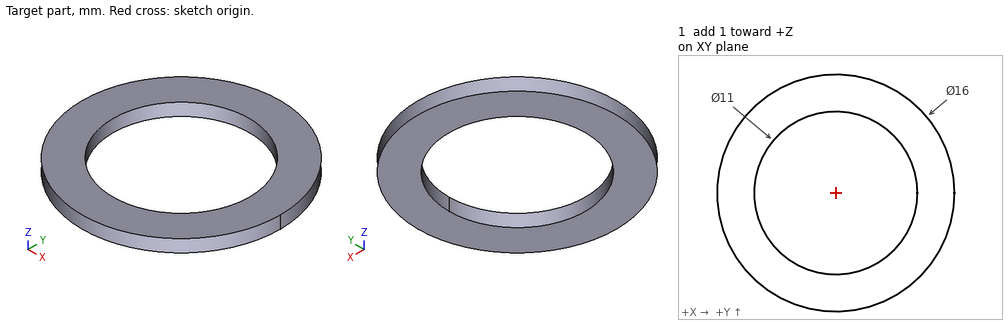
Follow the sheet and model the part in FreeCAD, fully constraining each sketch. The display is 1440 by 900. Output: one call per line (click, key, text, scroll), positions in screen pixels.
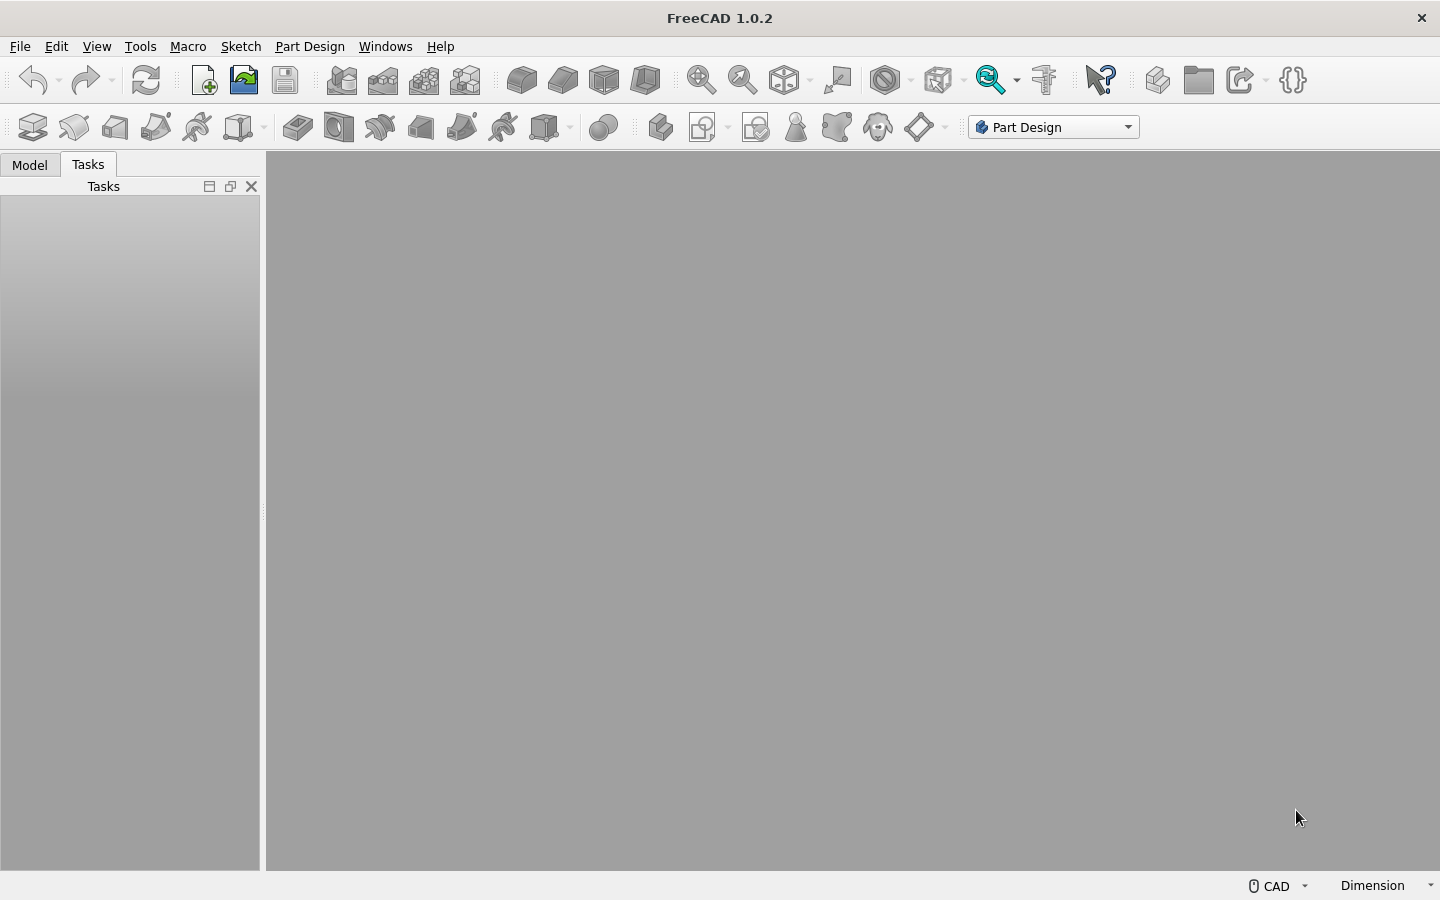
click(203, 80)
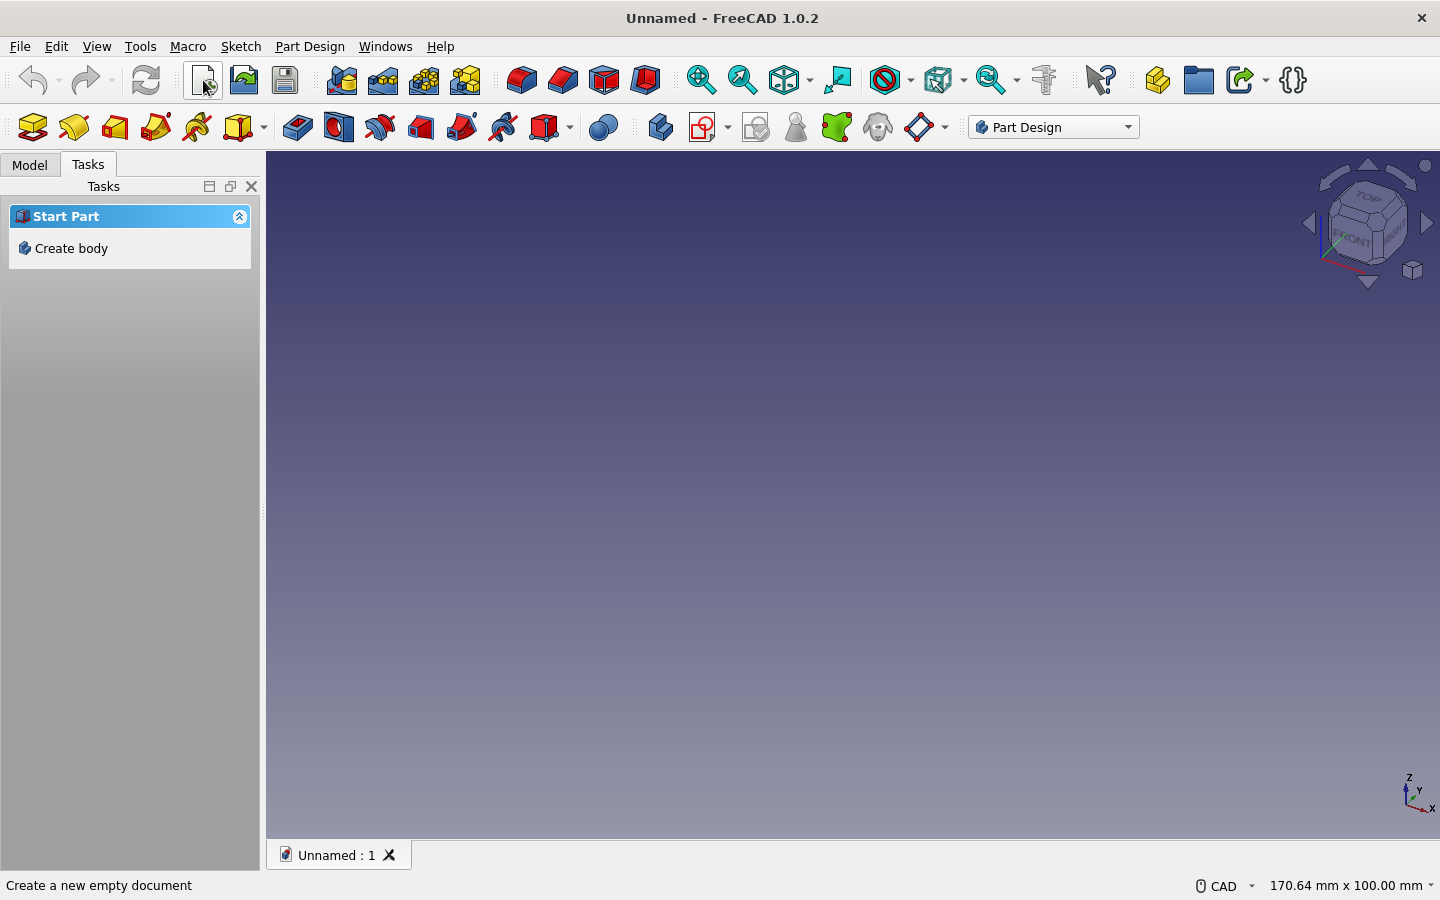
click(702, 128)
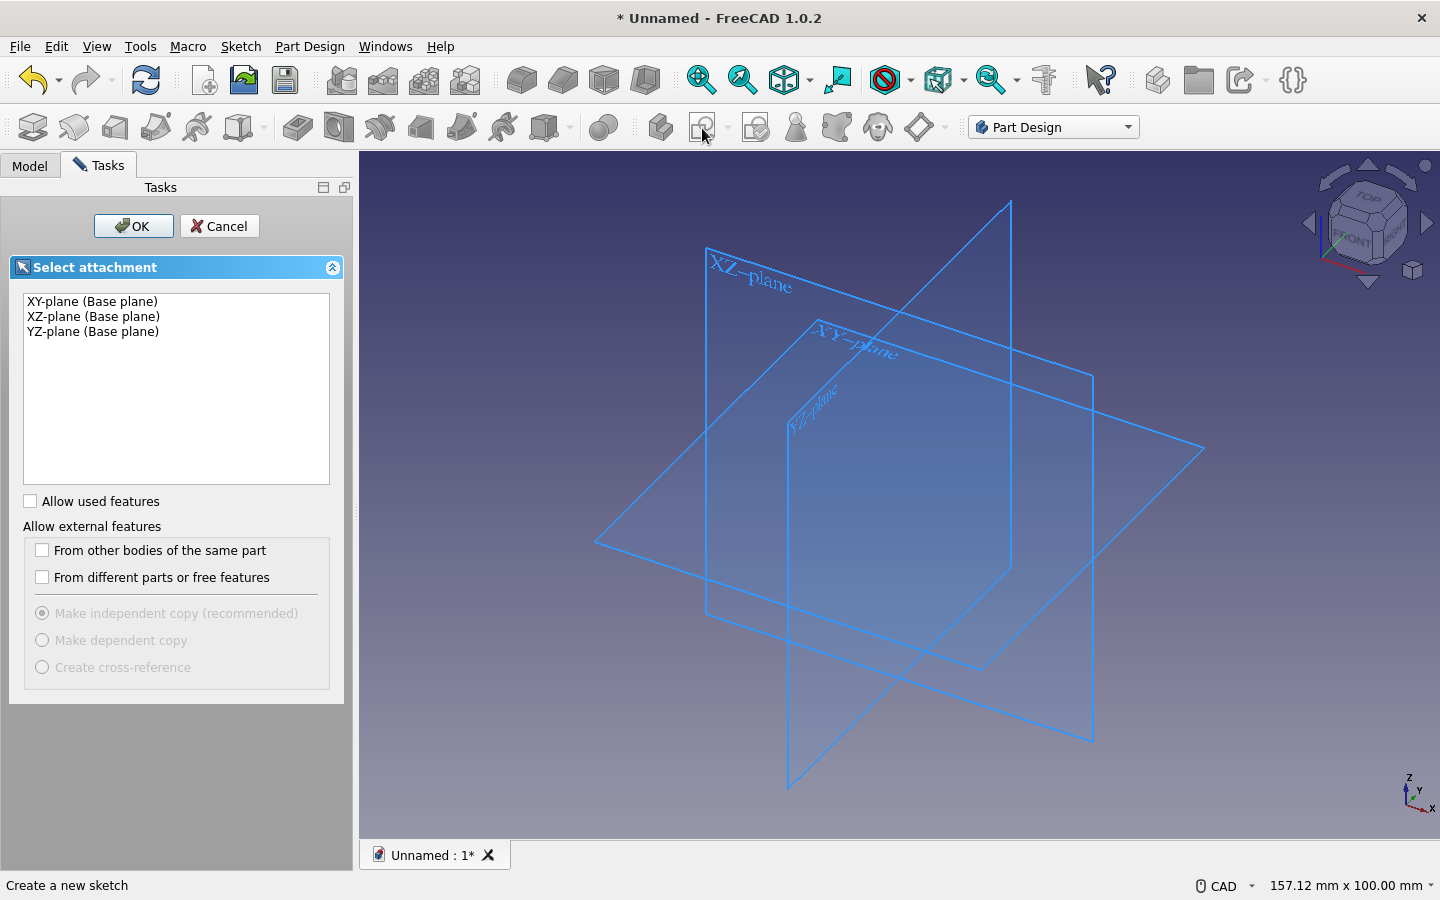
click(84, 302)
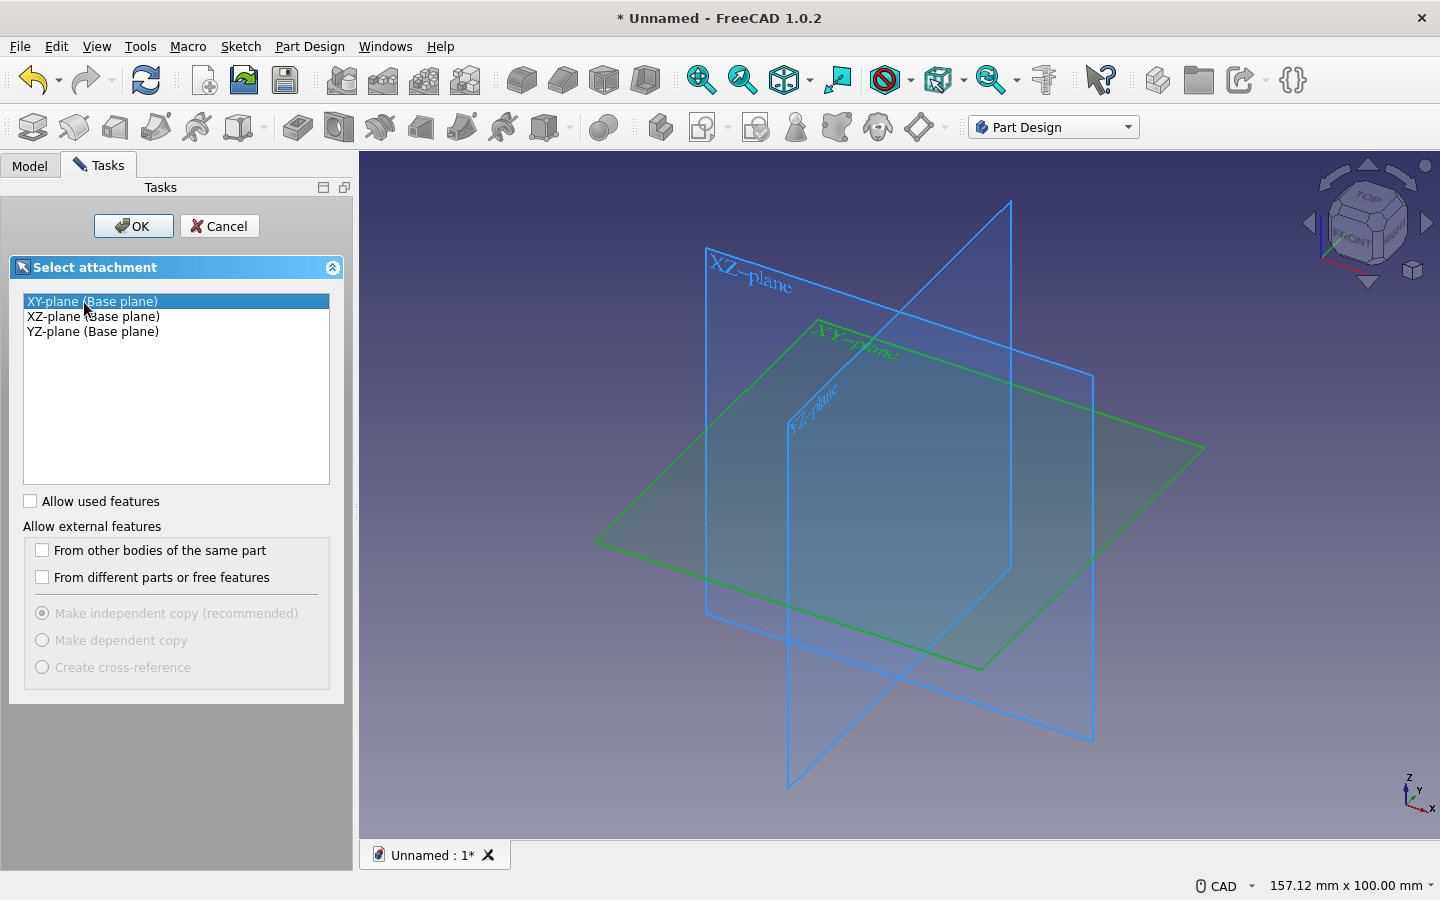
click(134, 226)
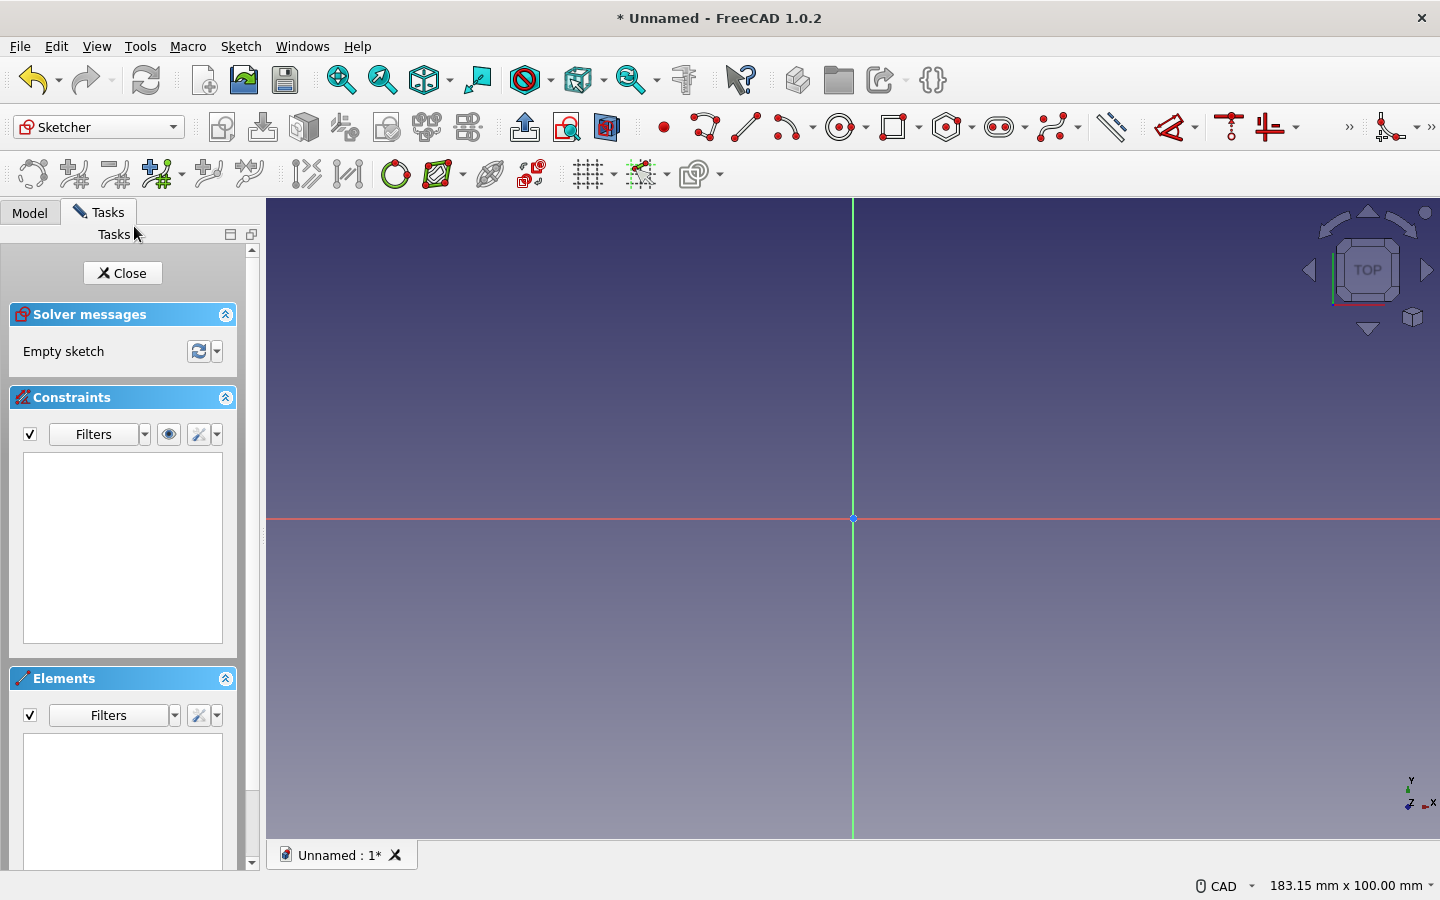
scroll(875, 518, up, 7)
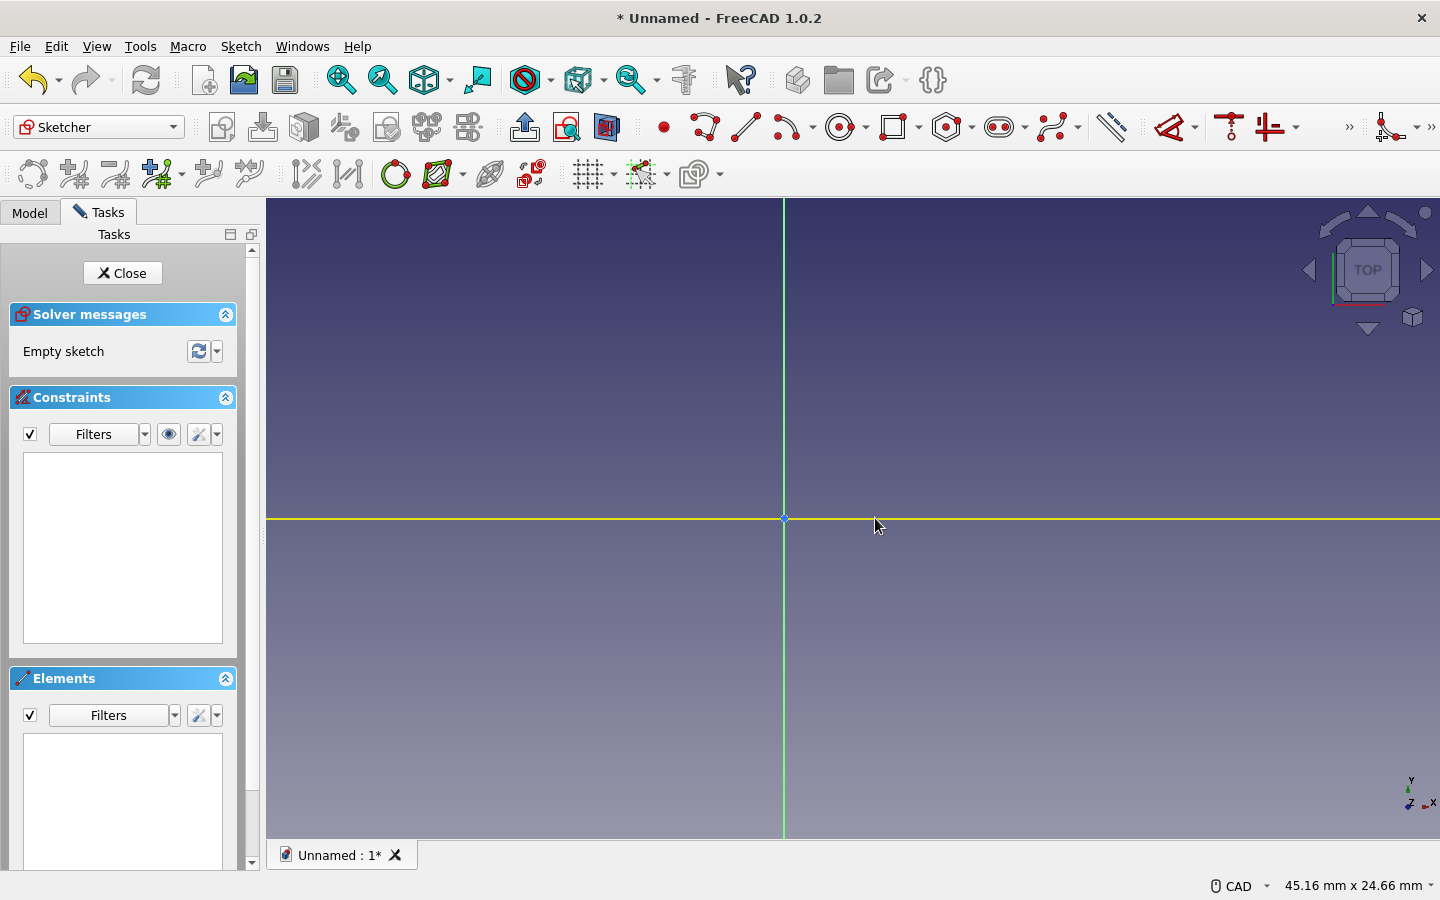
click(840, 128)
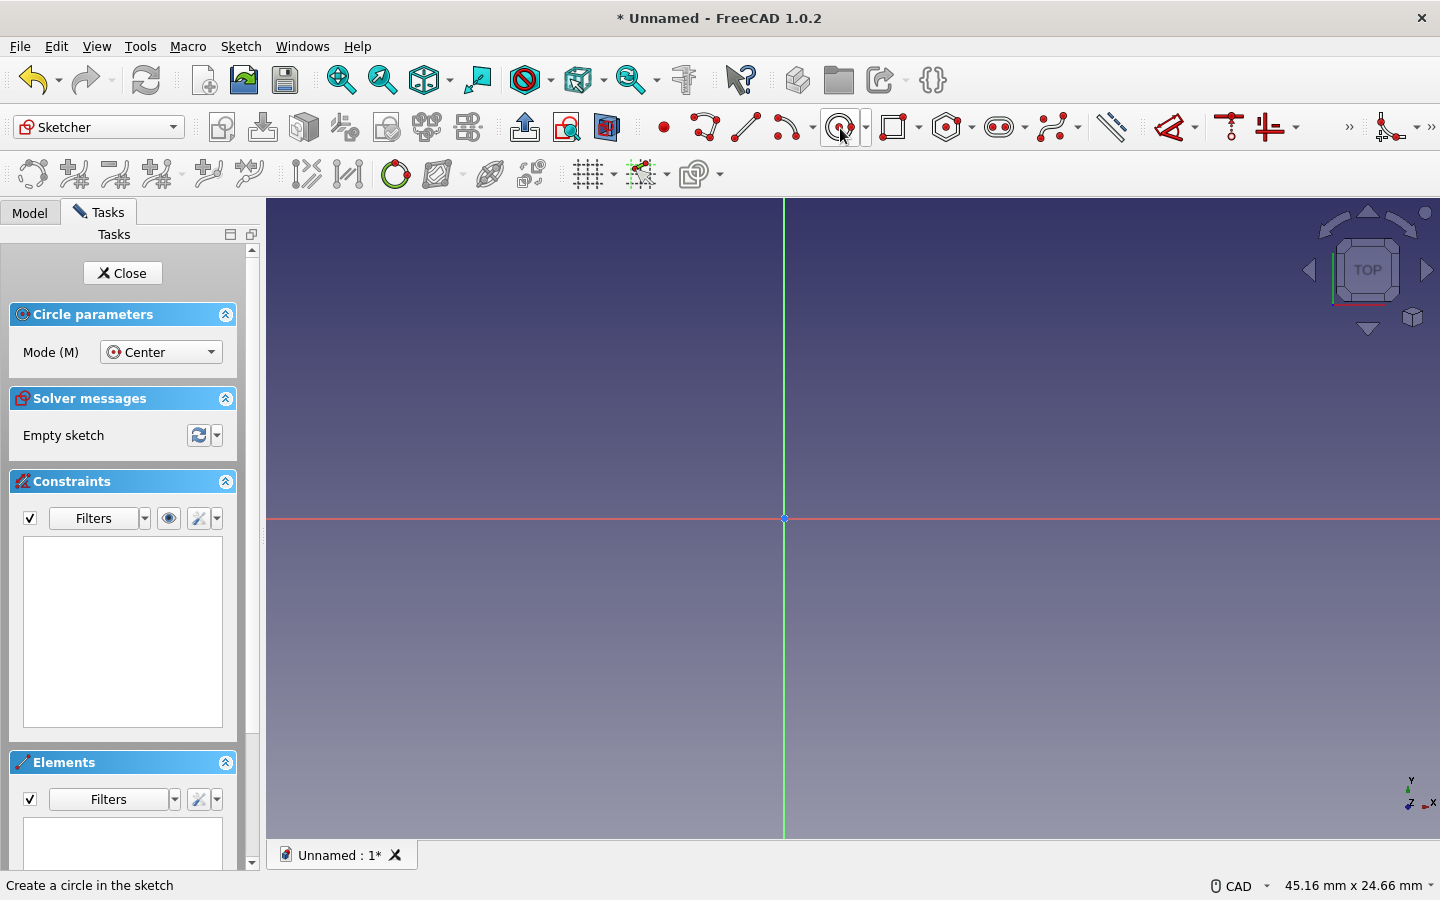
click(784, 518)
click(931, 371)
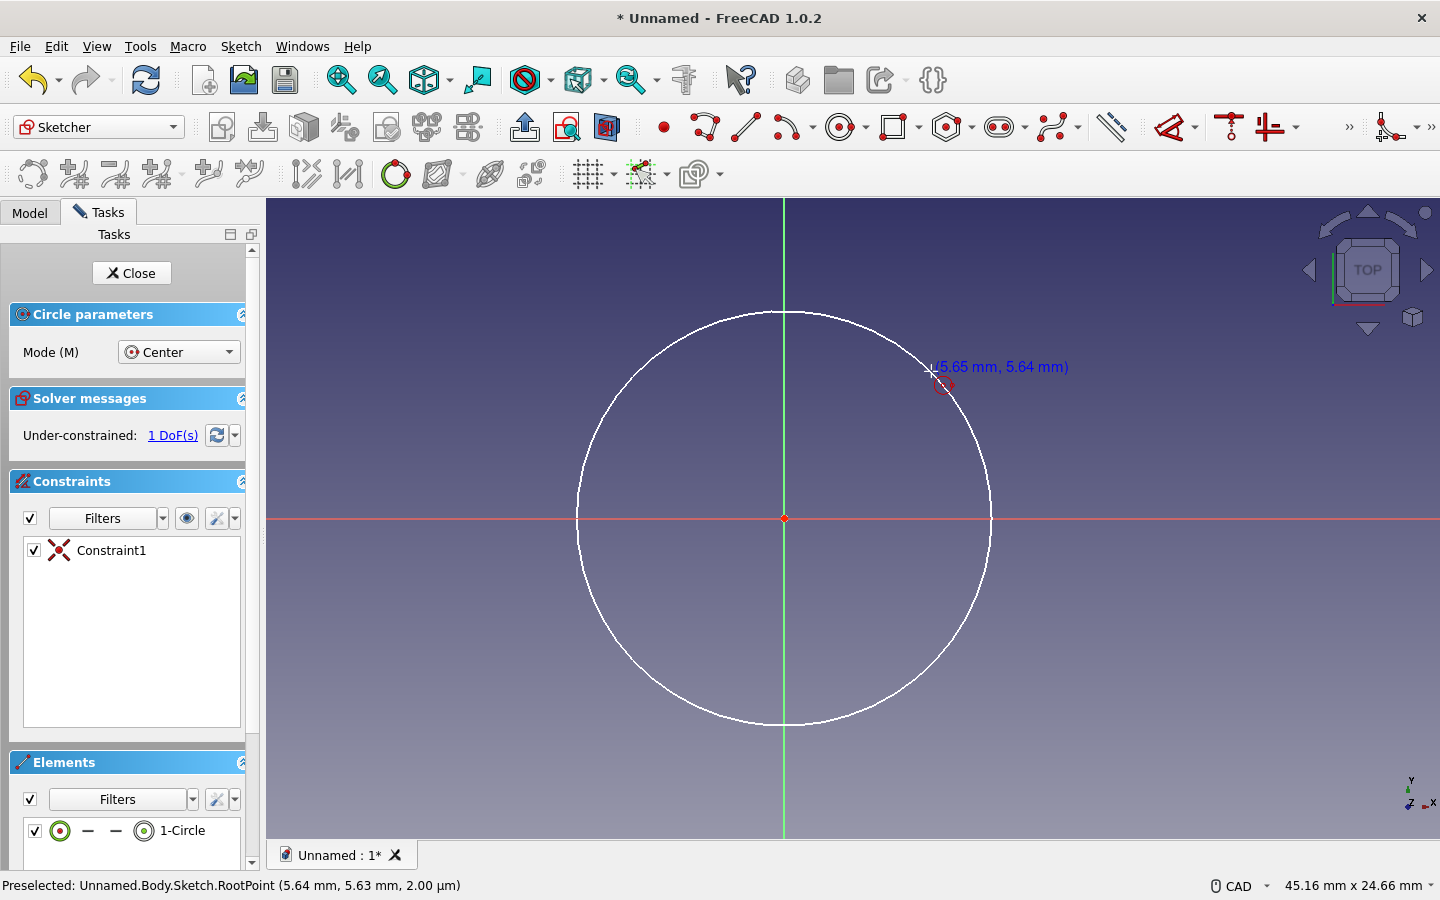
click(784, 518)
click(885, 417)
key(Escape)